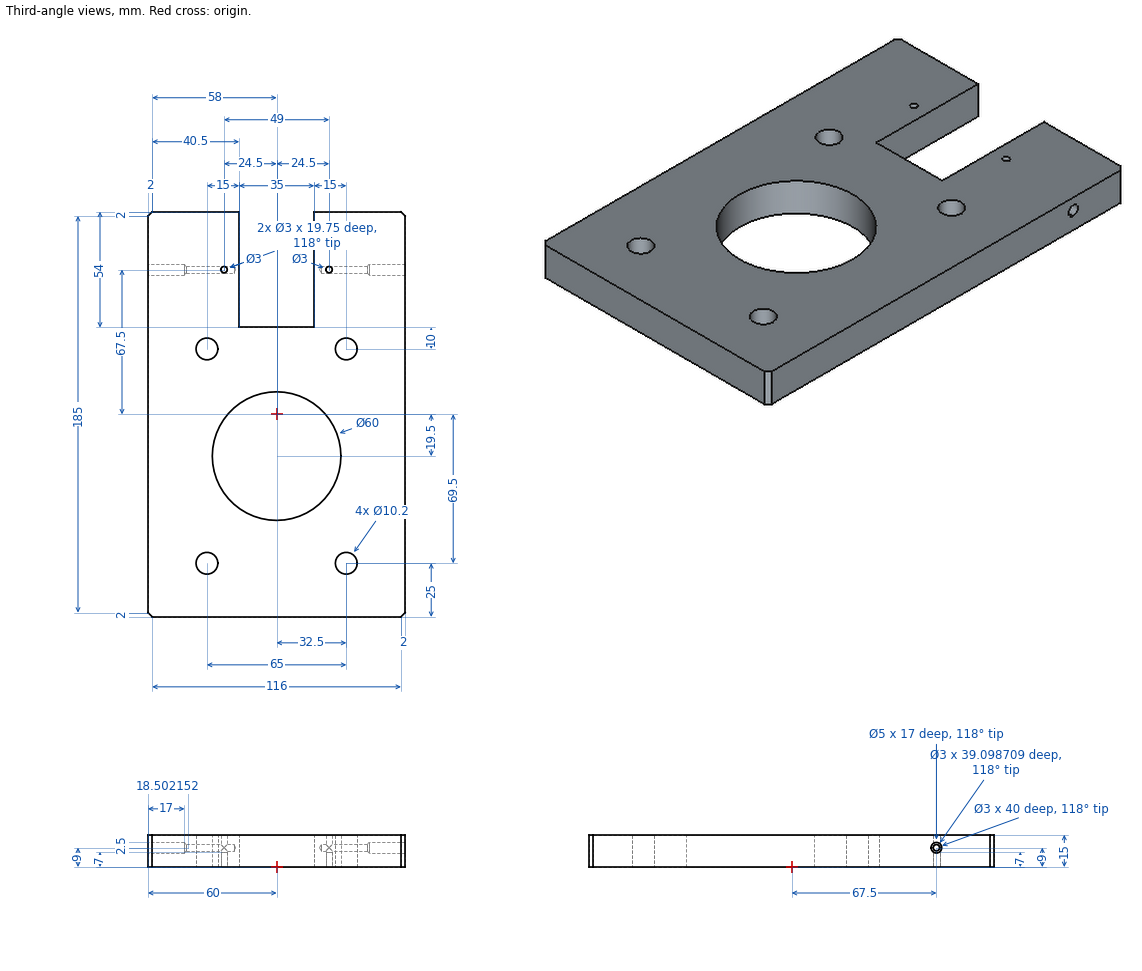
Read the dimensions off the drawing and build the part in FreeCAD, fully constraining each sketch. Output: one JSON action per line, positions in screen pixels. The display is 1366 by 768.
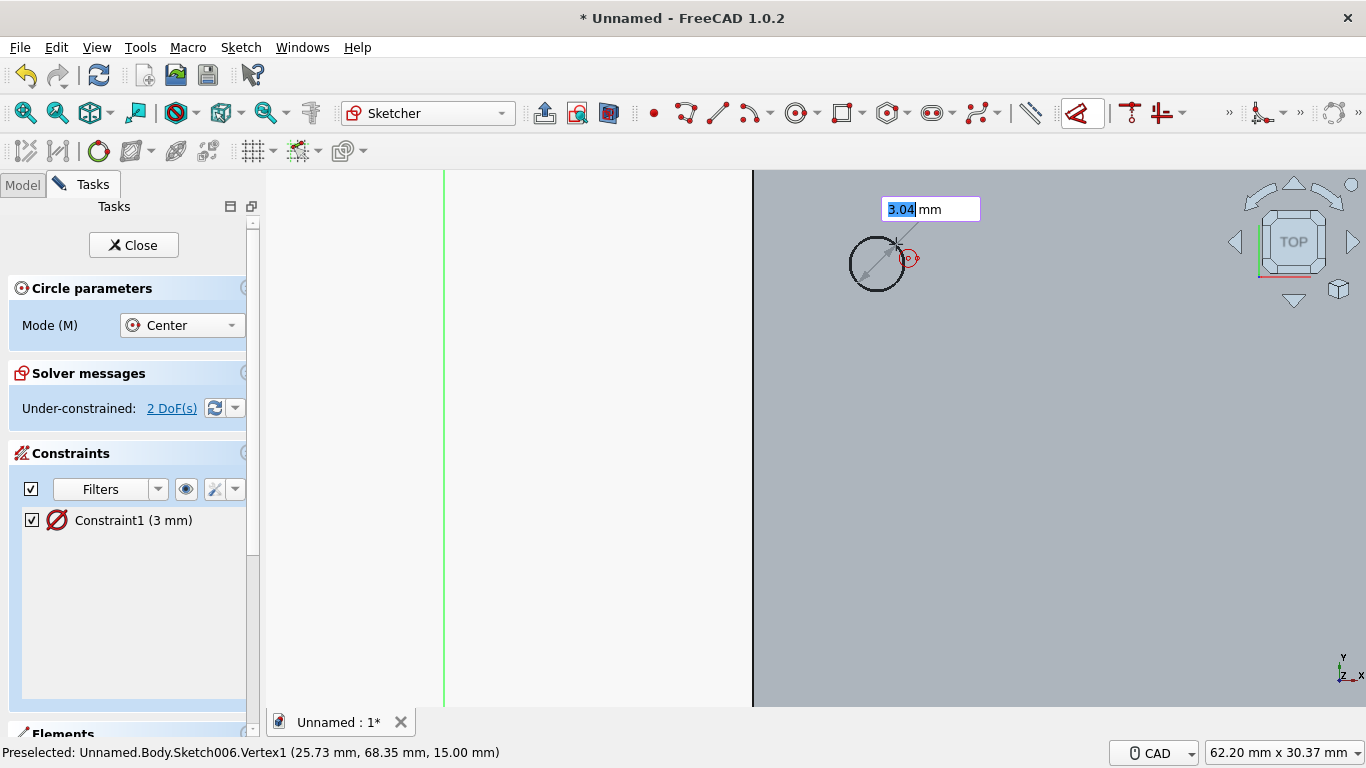
{"action": "type", "text": "3"}
{"action": "key", "text": "Return"}
{"action": "key", "text": "Escape"}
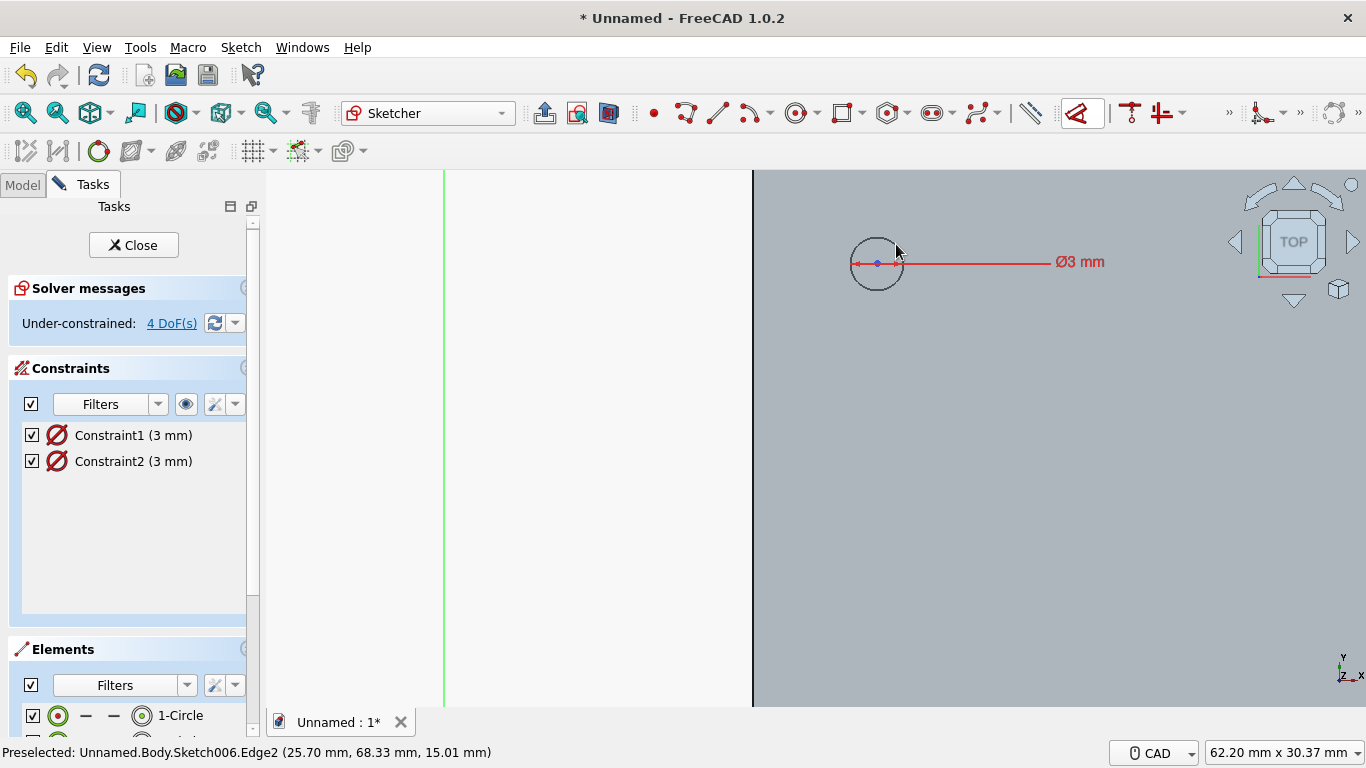
{"action": "scroll", "coordinate": [878, 263], "scroll_direction": "down", "scroll_amount": 6}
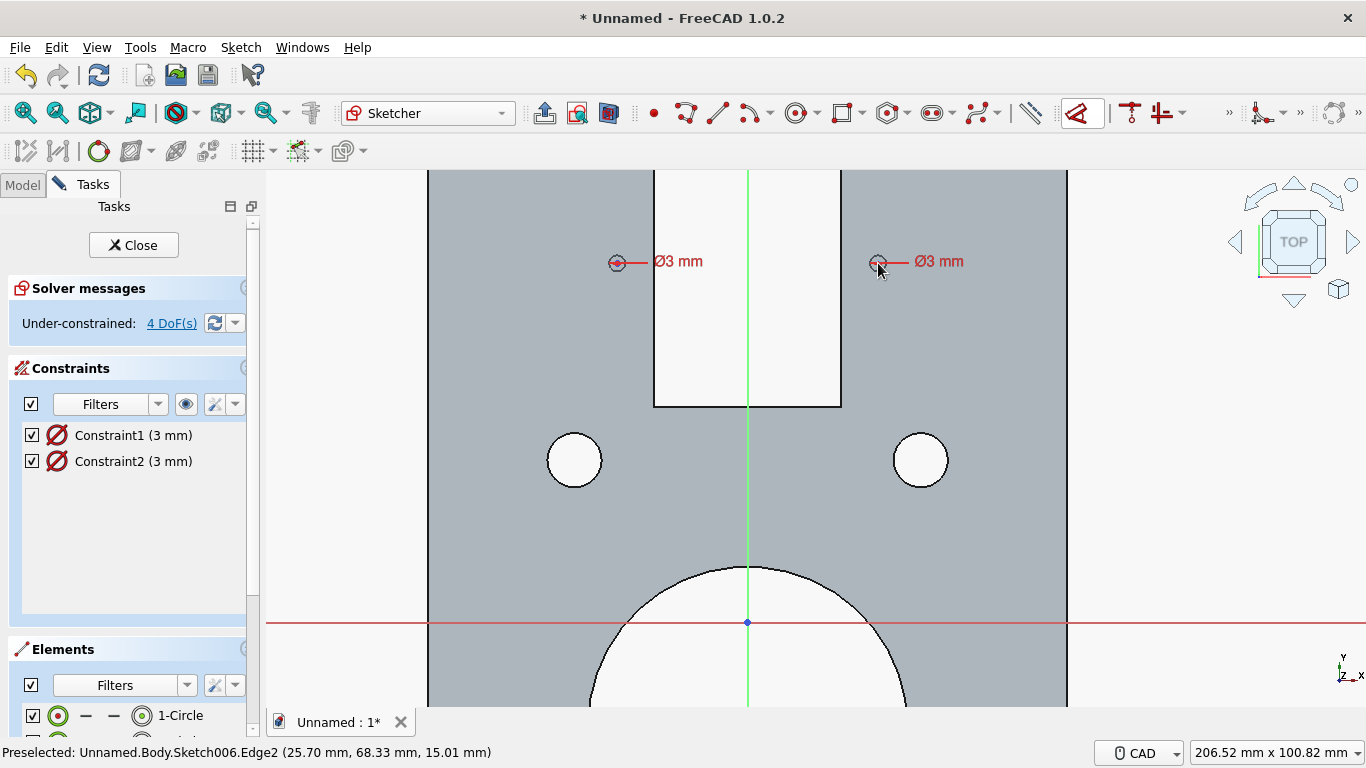
{"action": "left_click", "coordinate": [617, 263]}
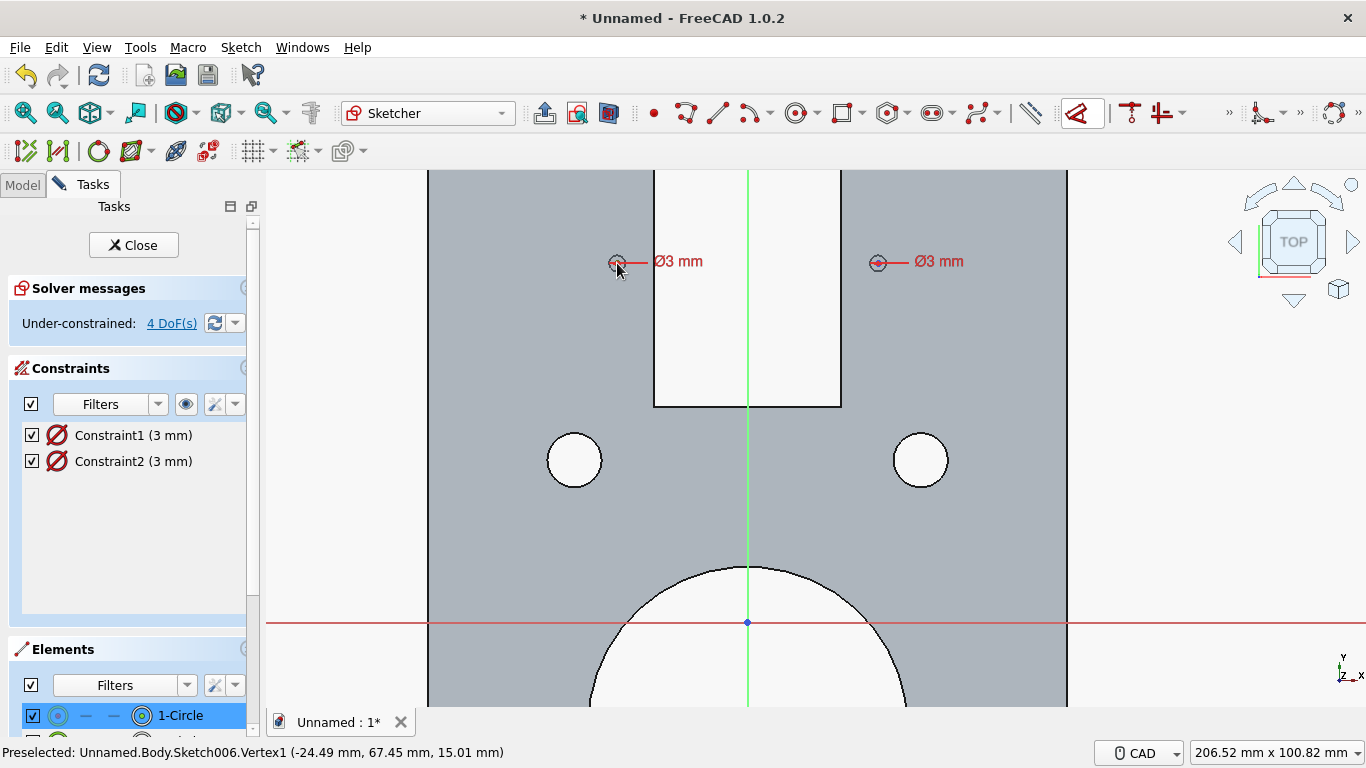
{"action": "left_click", "coordinate": [878, 263]}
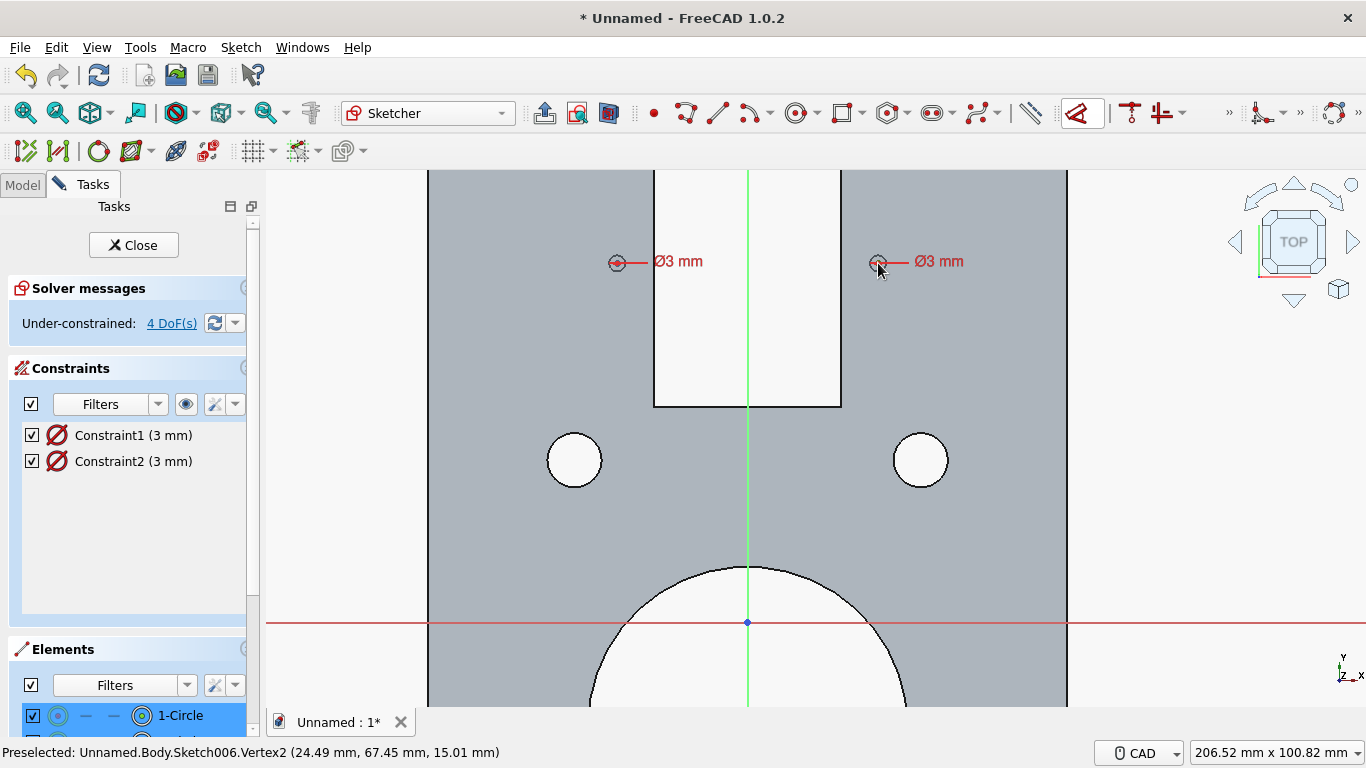
{"action": "left_click", "coordinate": [1098, 114]}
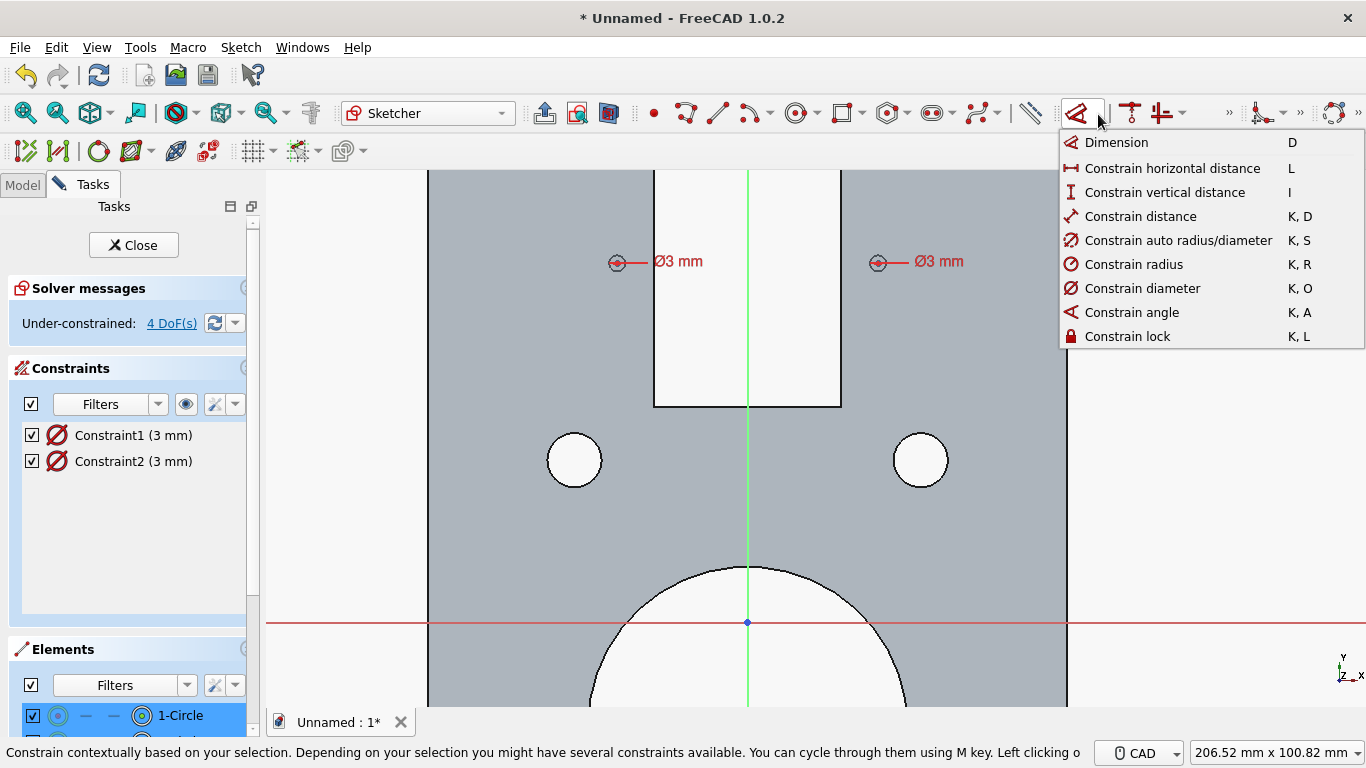
{"action": "left_click", "coordinate": [1212, 168]}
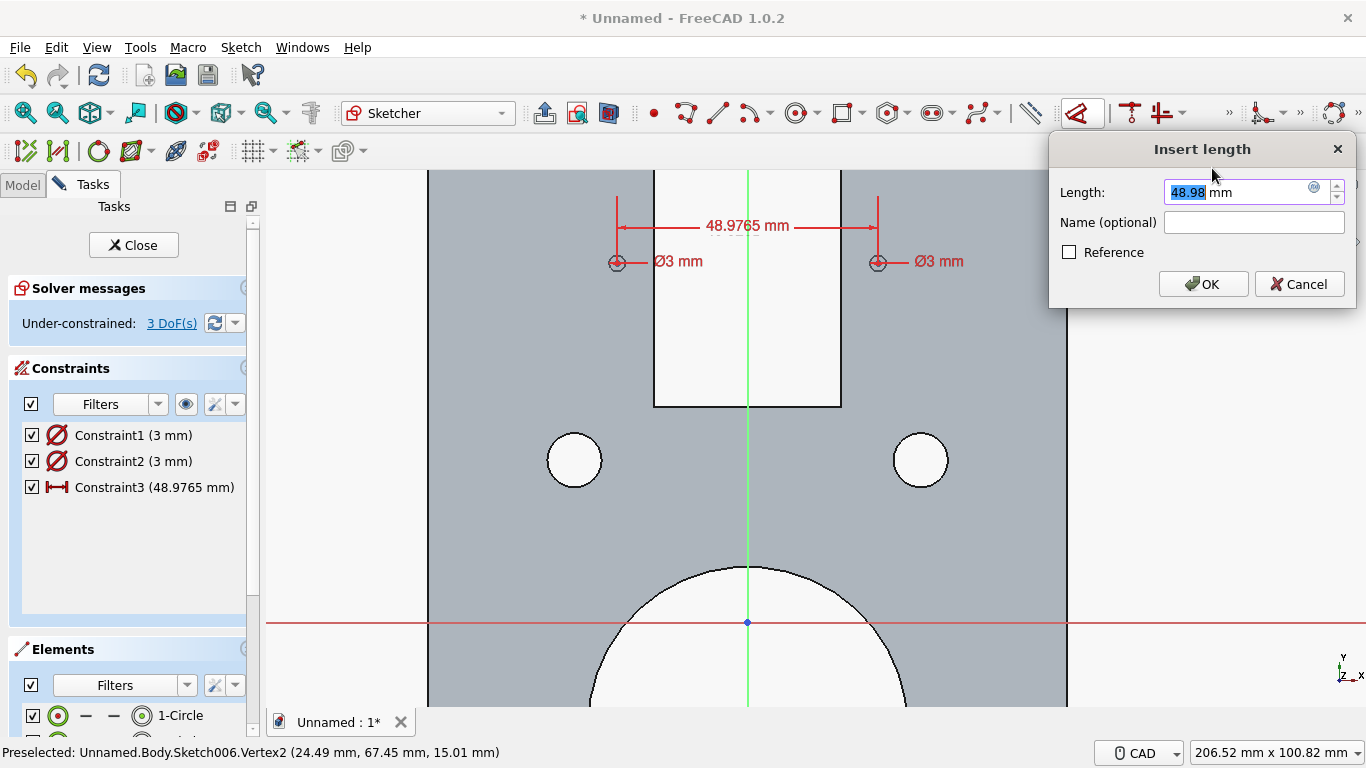
{"action": "type", "text": "49"}
{"action": "key", "text": "Return"}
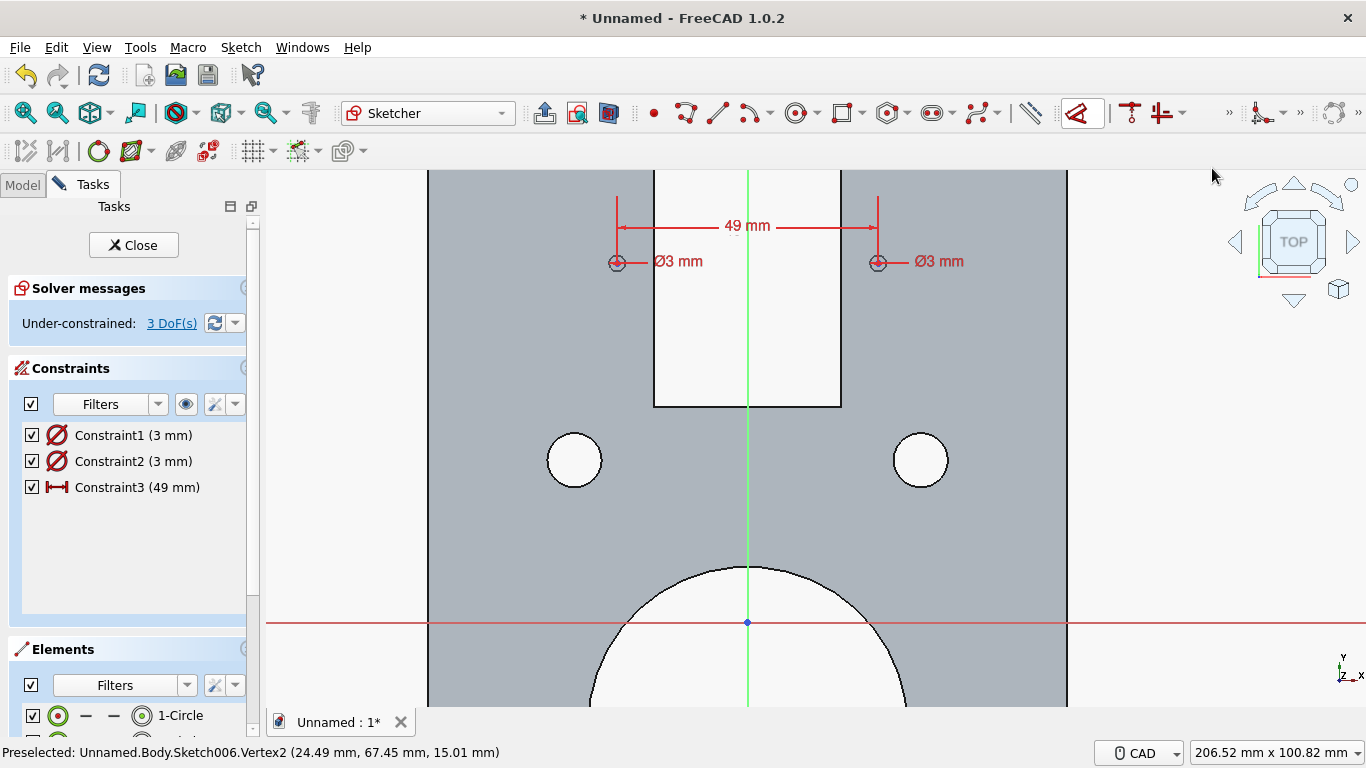
{"action": "left_click", "coordinate": [617, 263]}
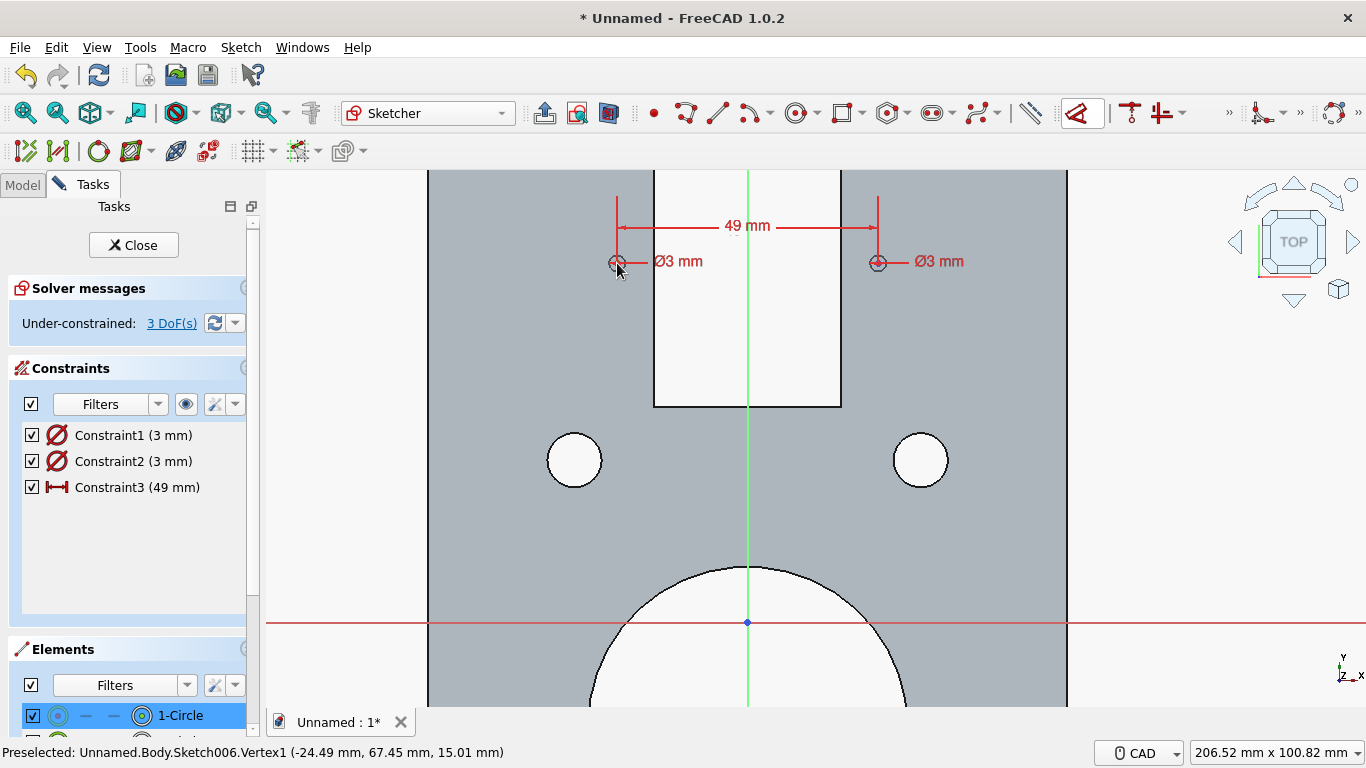
{"action": "left_click", "coordinate": [1098, 114]}